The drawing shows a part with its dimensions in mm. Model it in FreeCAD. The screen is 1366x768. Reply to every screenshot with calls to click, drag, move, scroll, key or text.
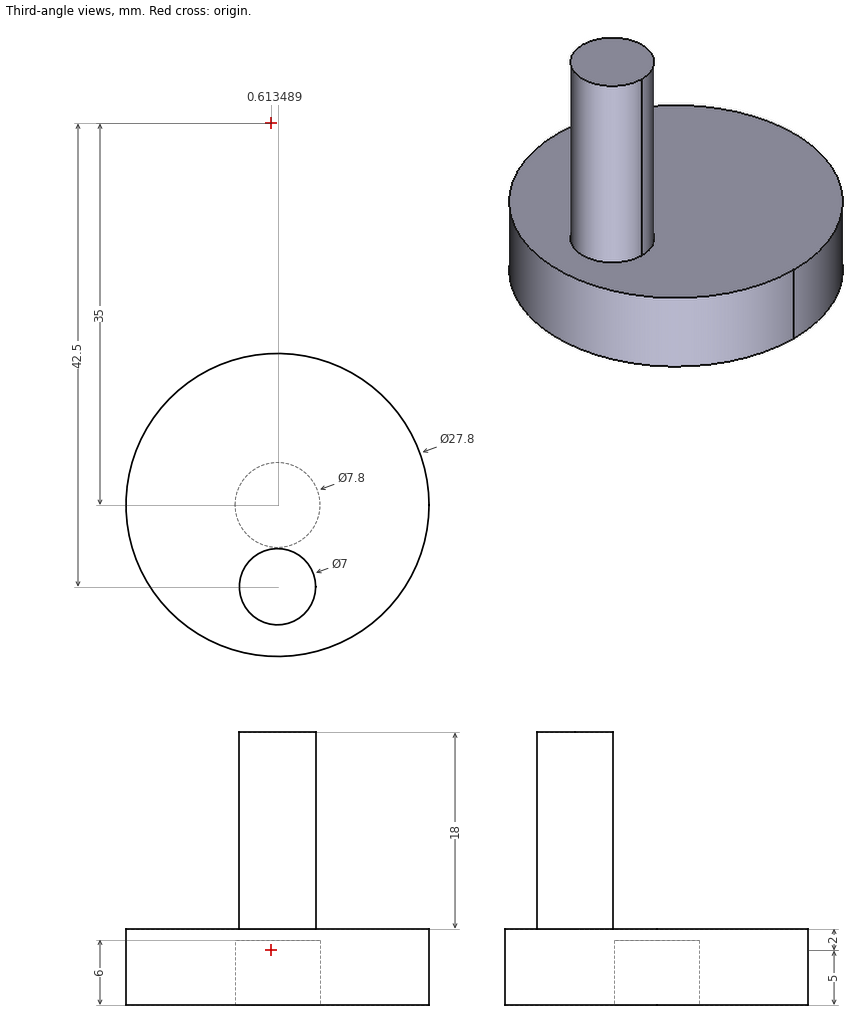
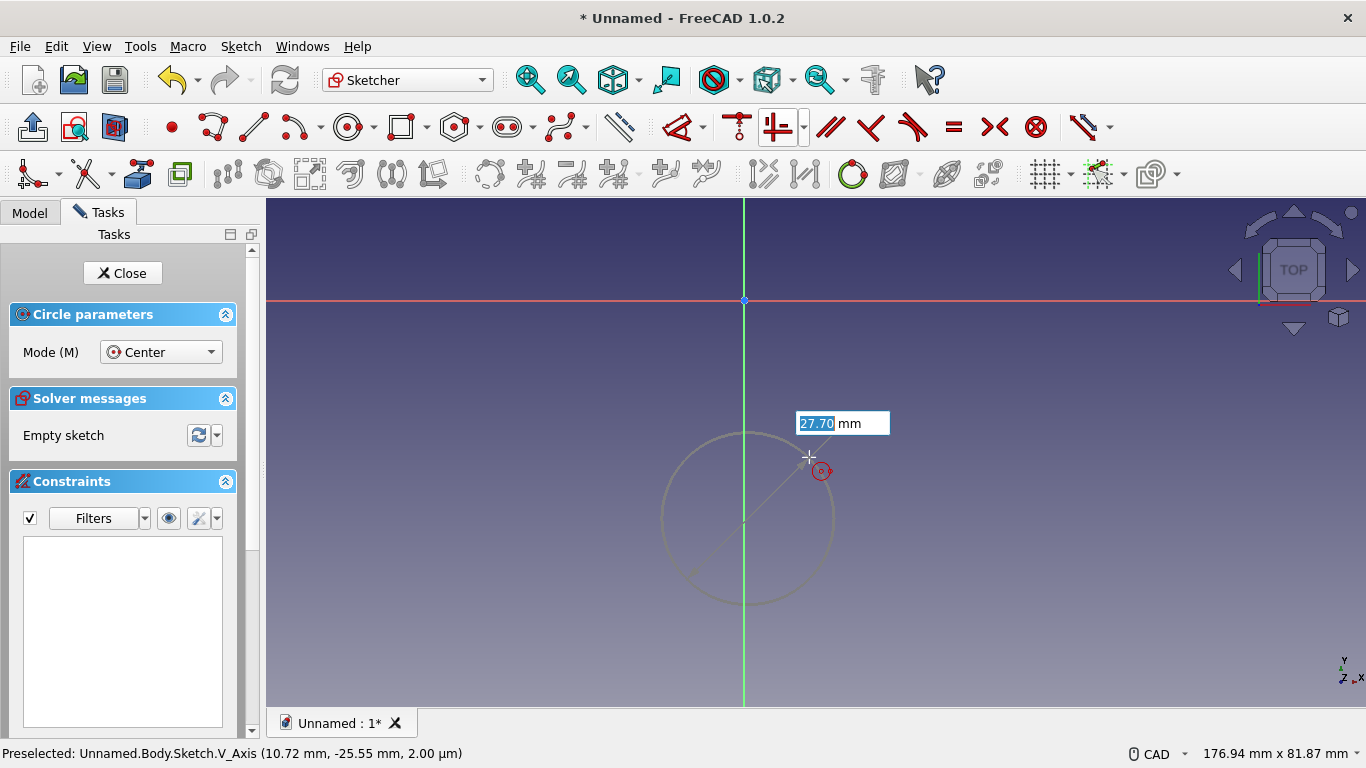
text(27.8)
key(Return)
key(Escape)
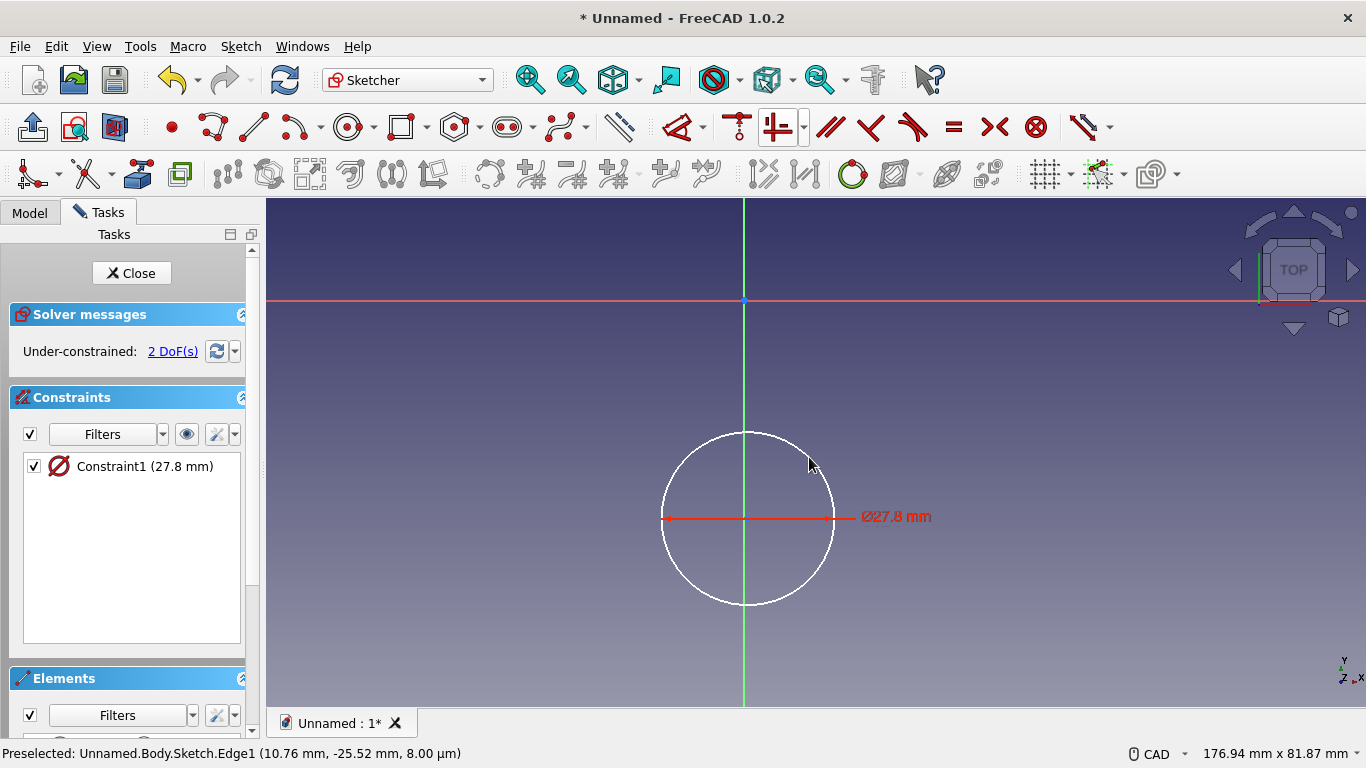
click(676, 128)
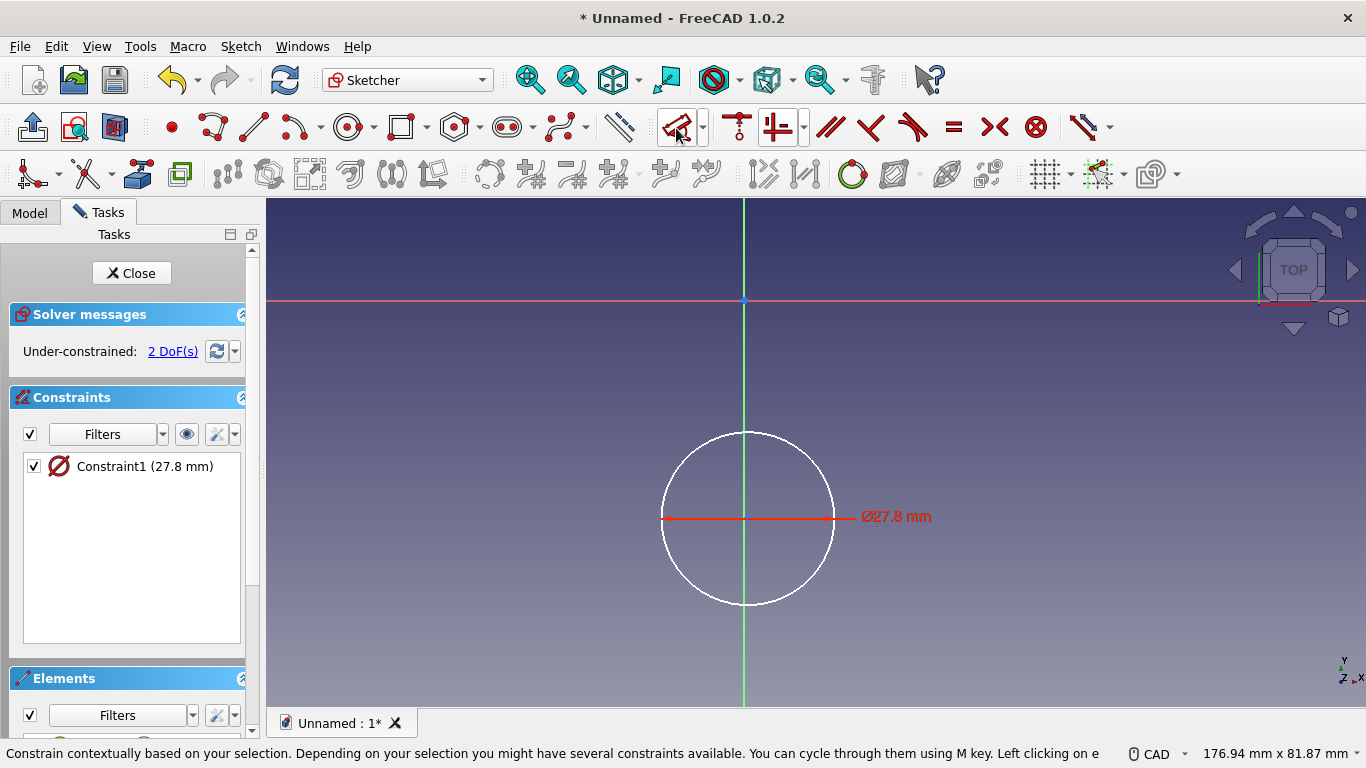
click(748, 519)
click(710, 410)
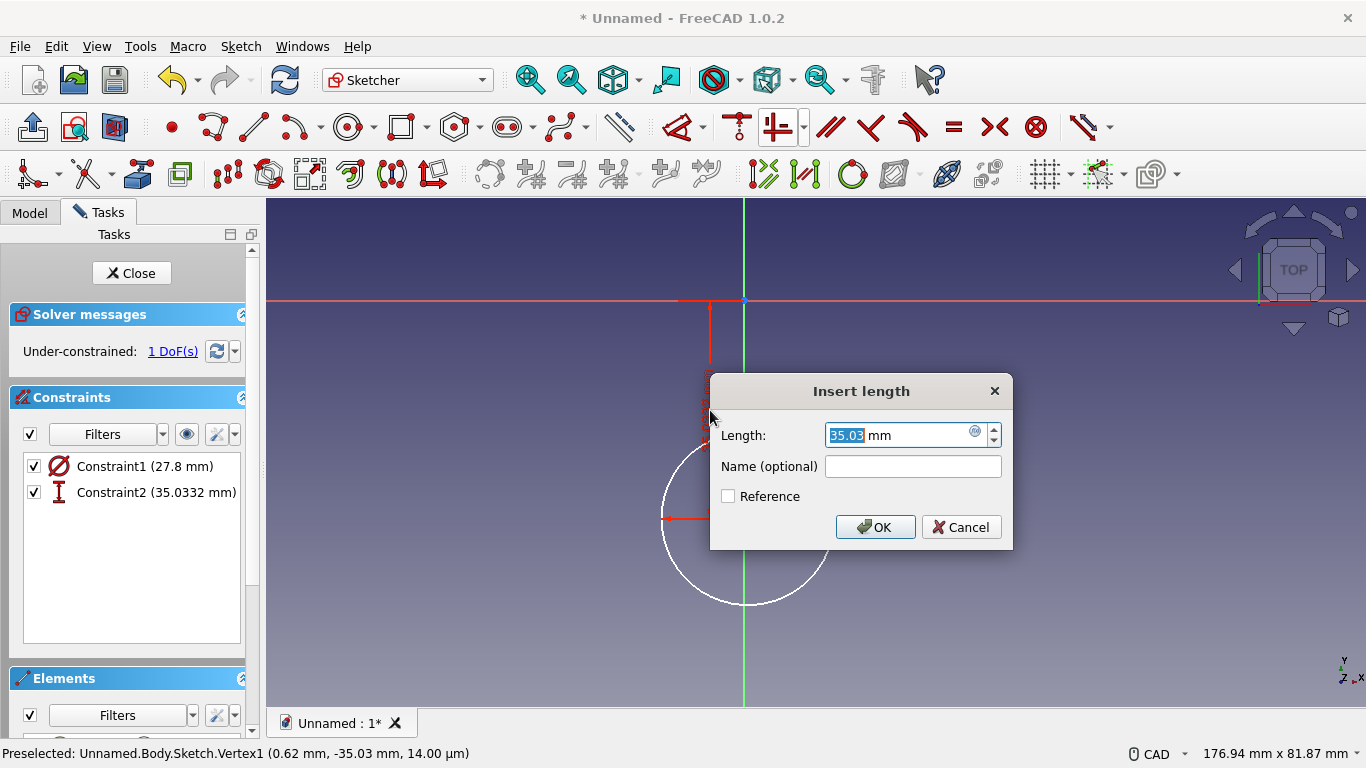
text(35)
key(Return)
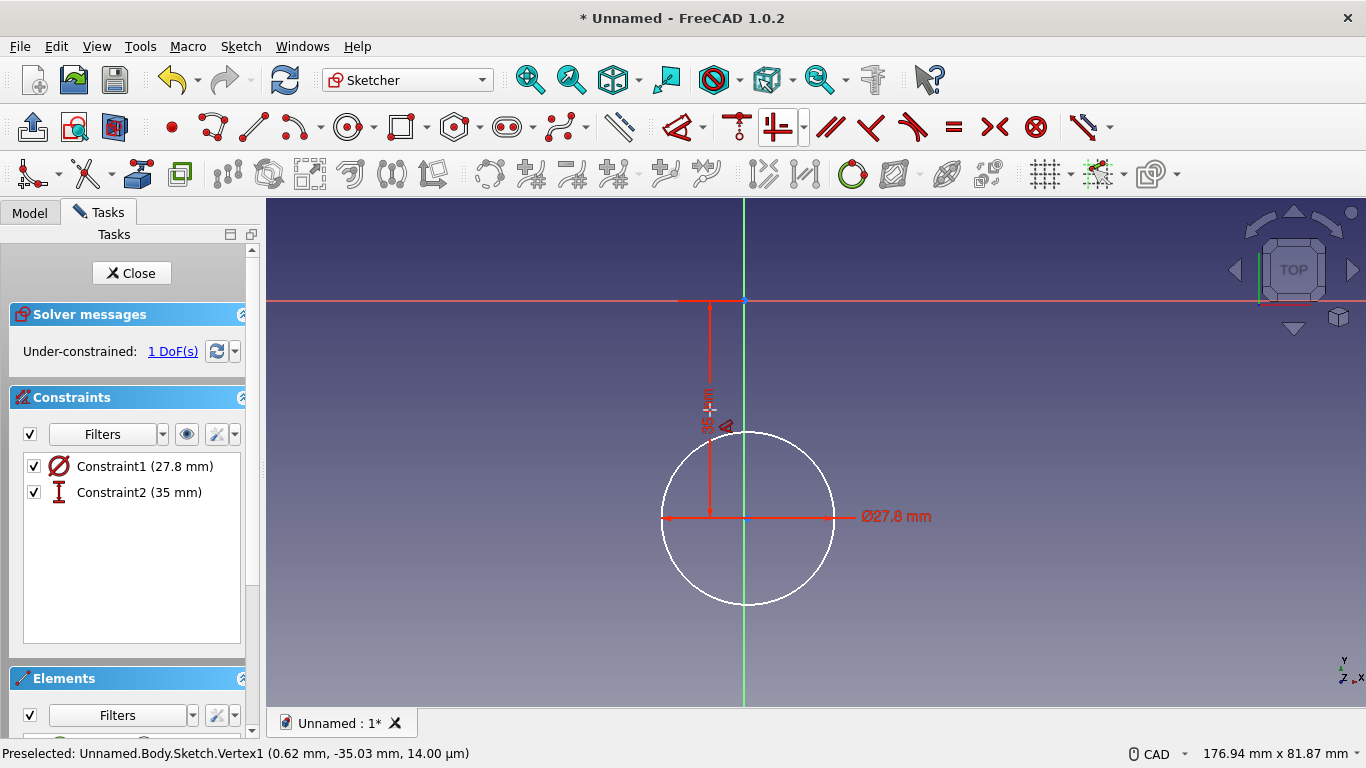
scroll(748, 518, up, 12)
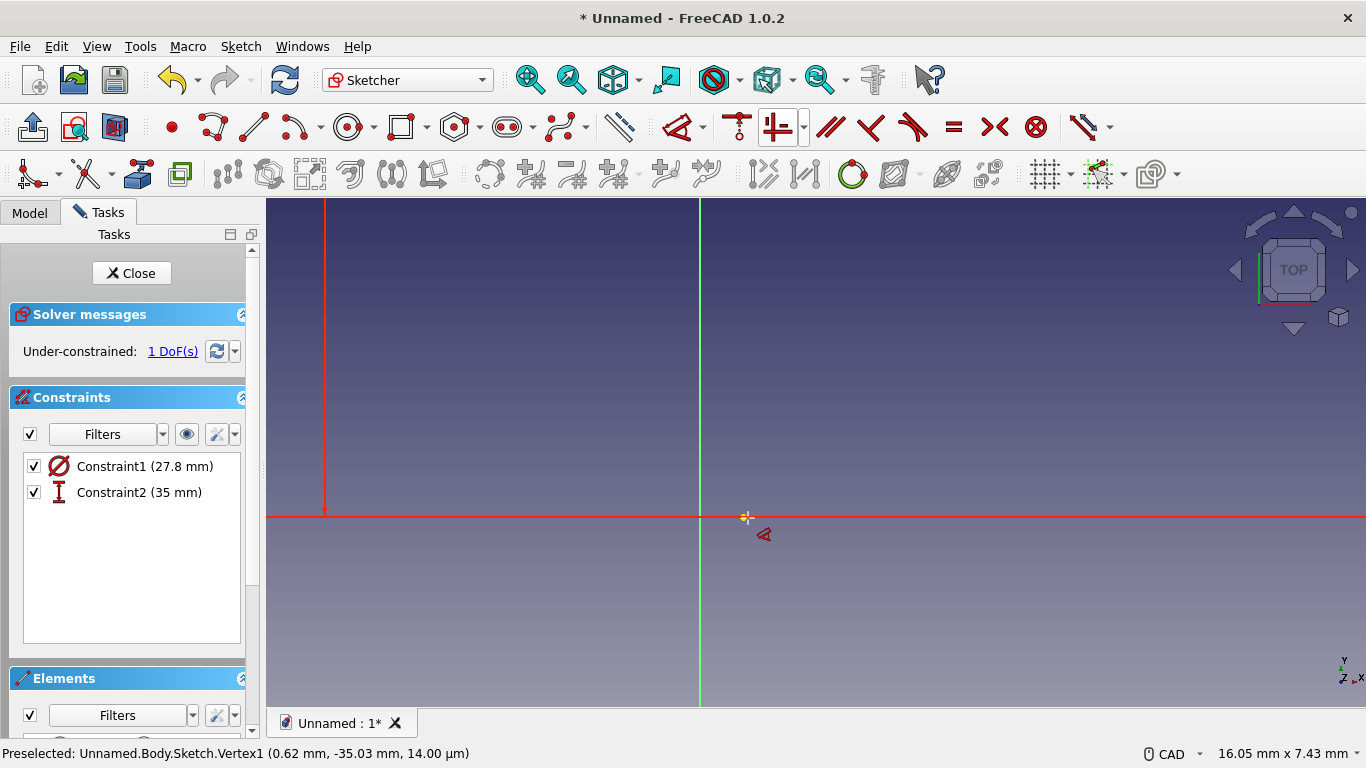
click(743, 517)
click(722, 551)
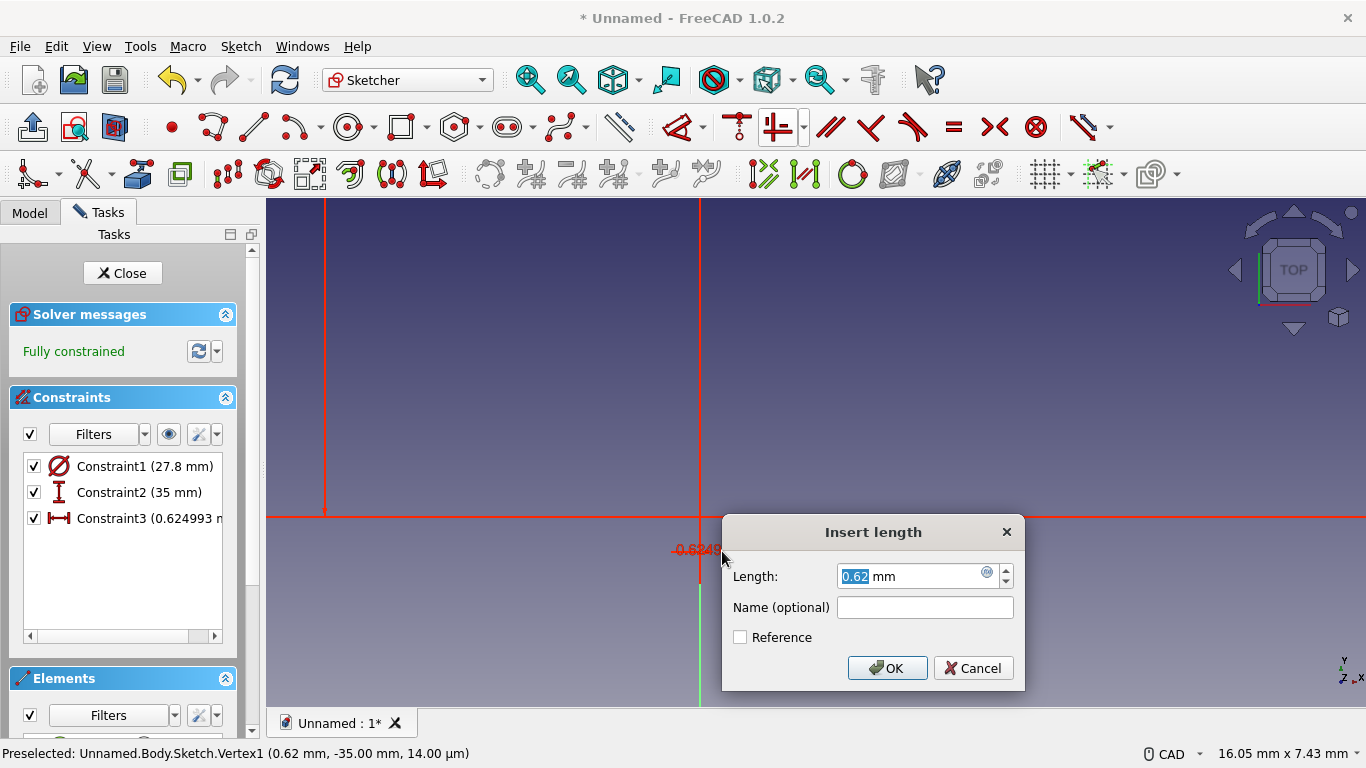
text(0.613489)
key(Return)
key(Escape)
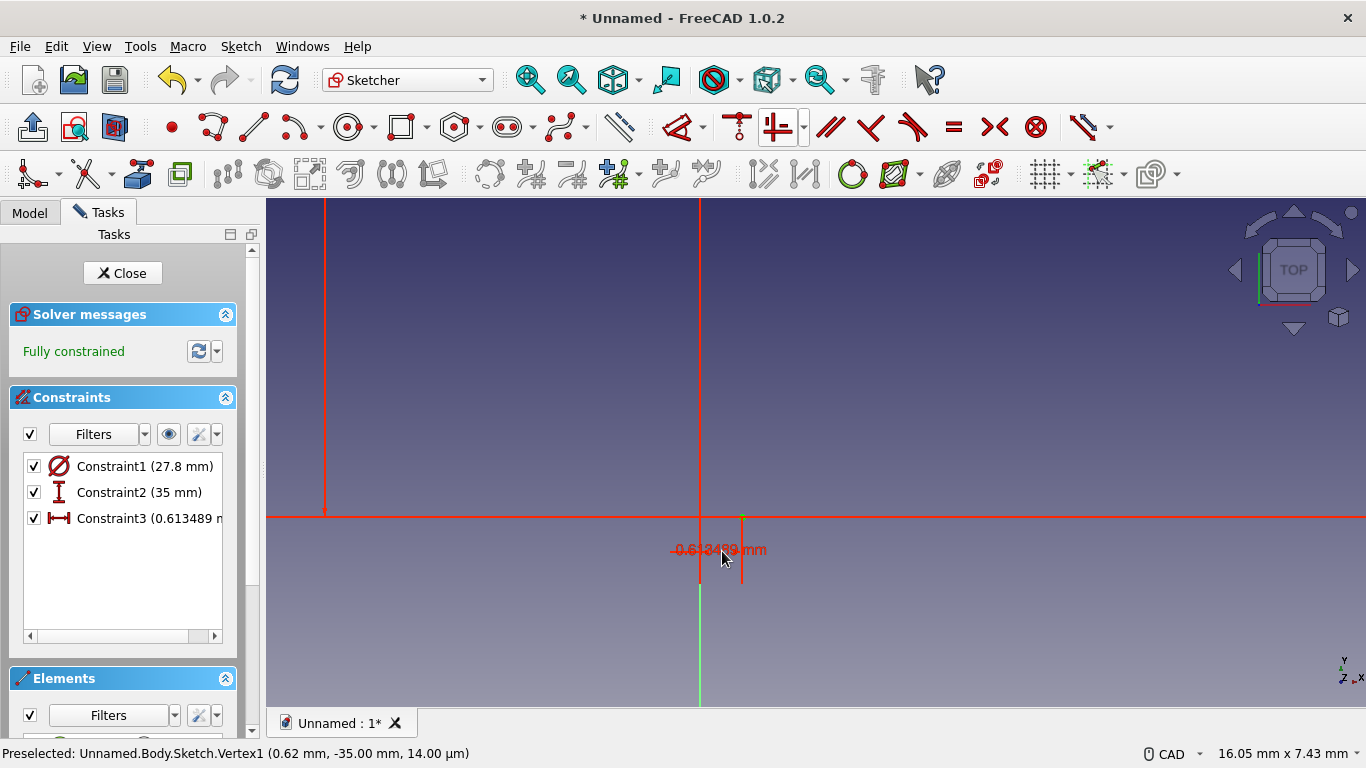
click(123, 273)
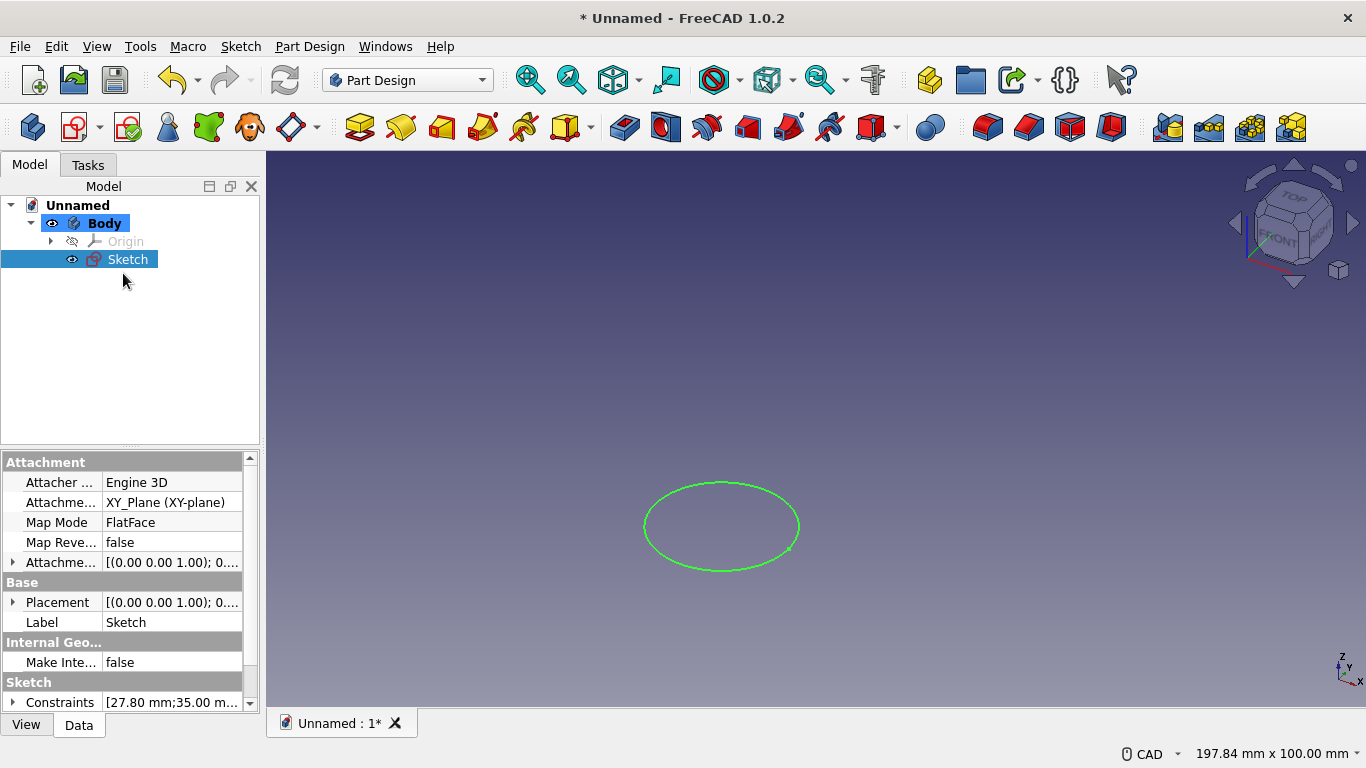
click(360, 128)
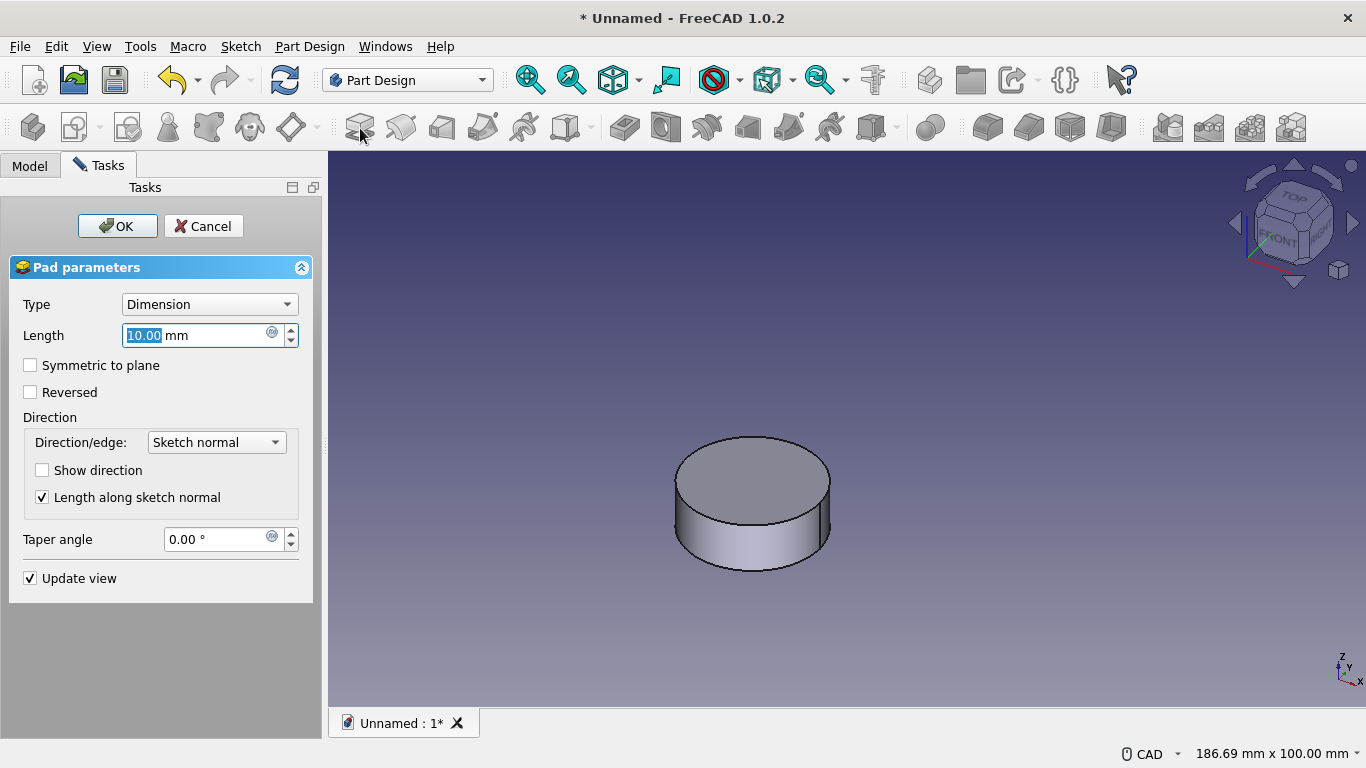
click(210, 304)